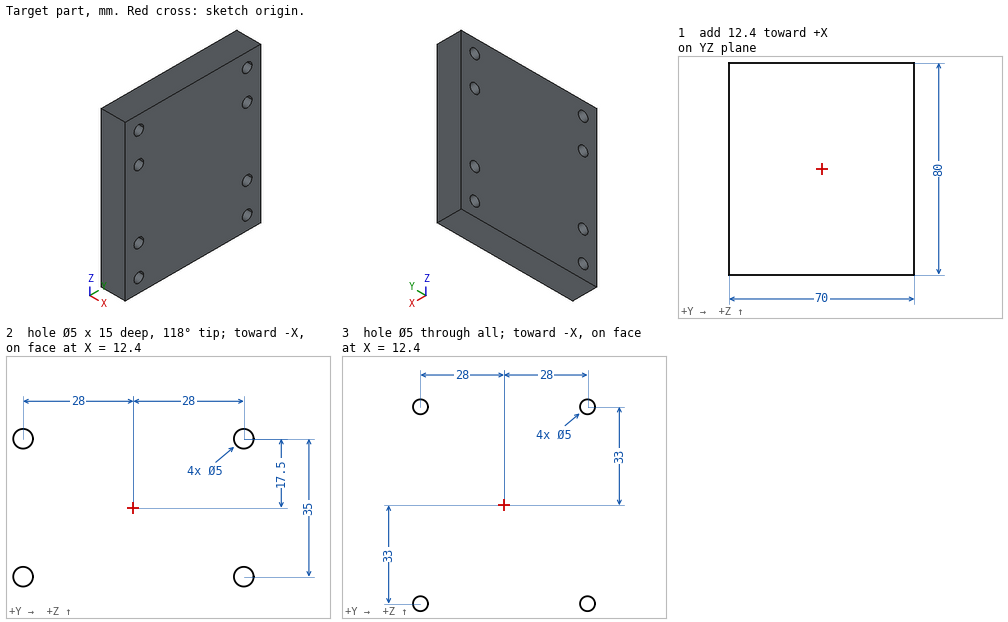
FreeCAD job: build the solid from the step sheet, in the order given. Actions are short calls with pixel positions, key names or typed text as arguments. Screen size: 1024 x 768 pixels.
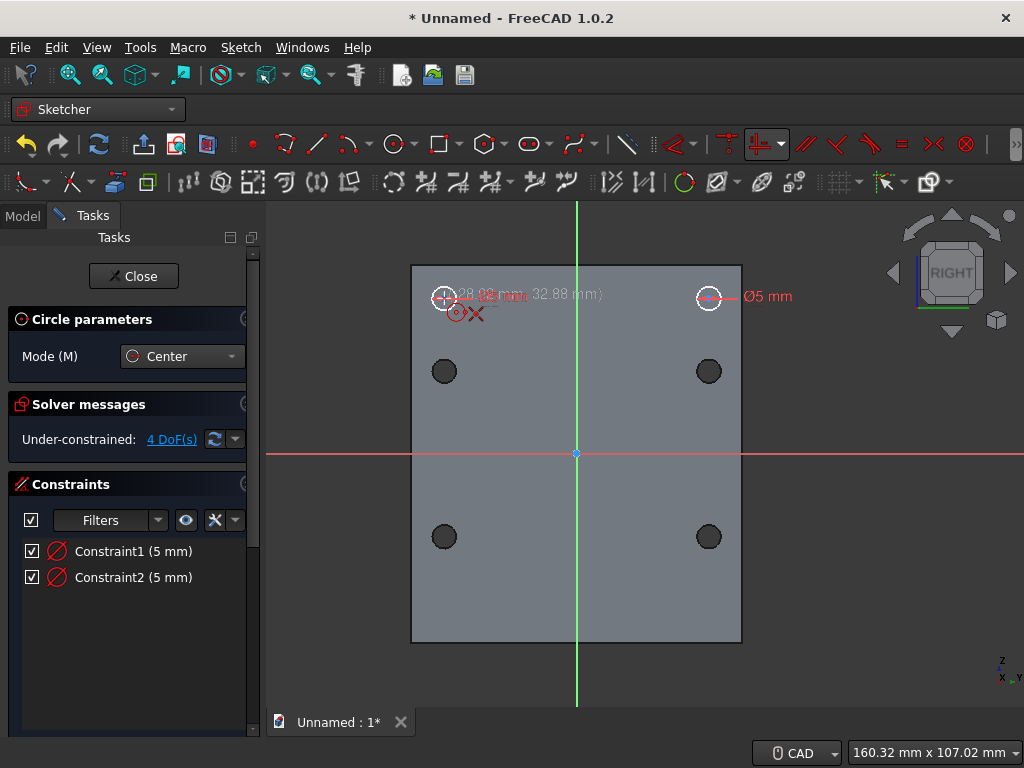
scroll(444, 610, up, 4)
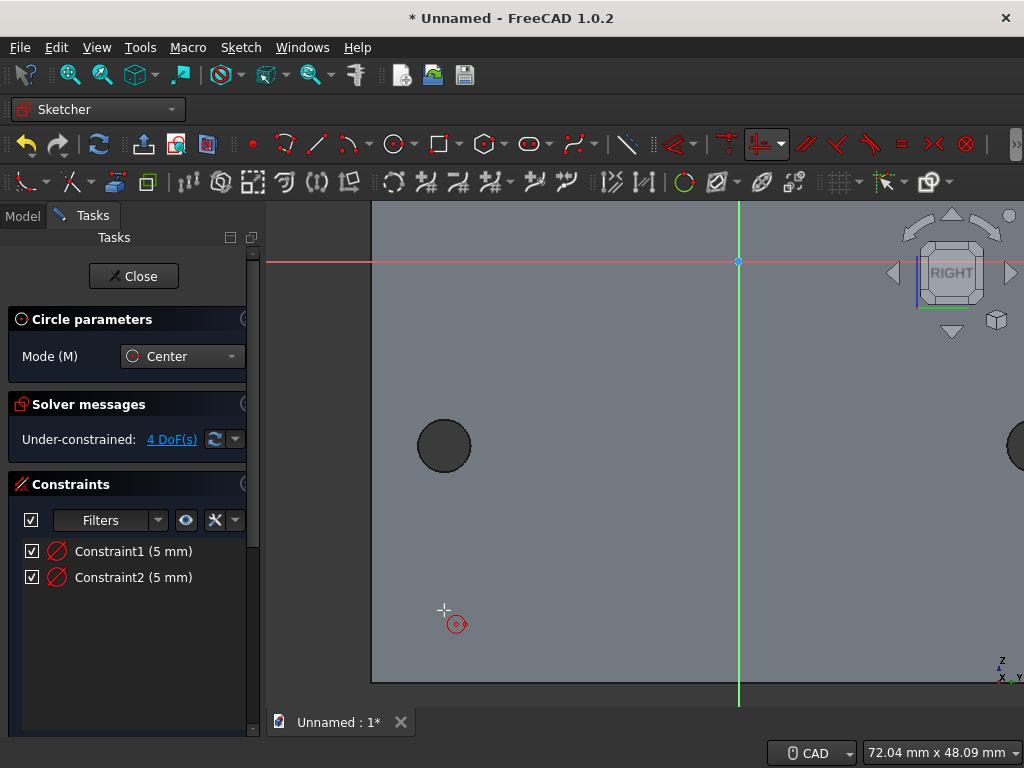
click(444, 609)
move(463, 590)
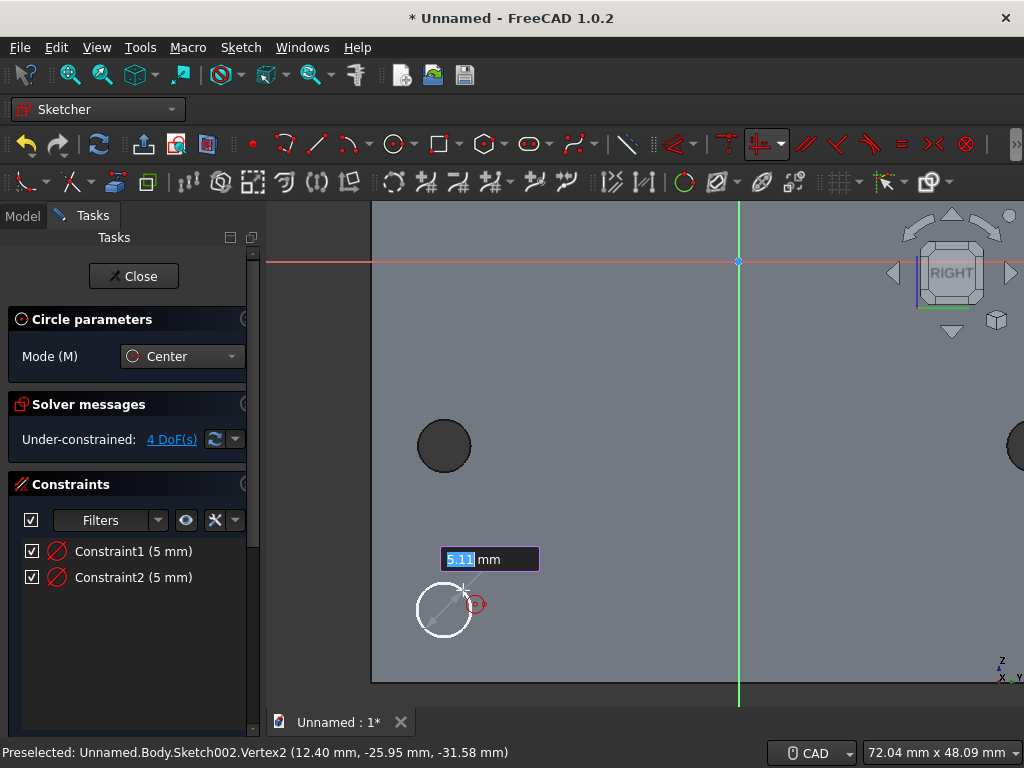
text(5)
key(Return)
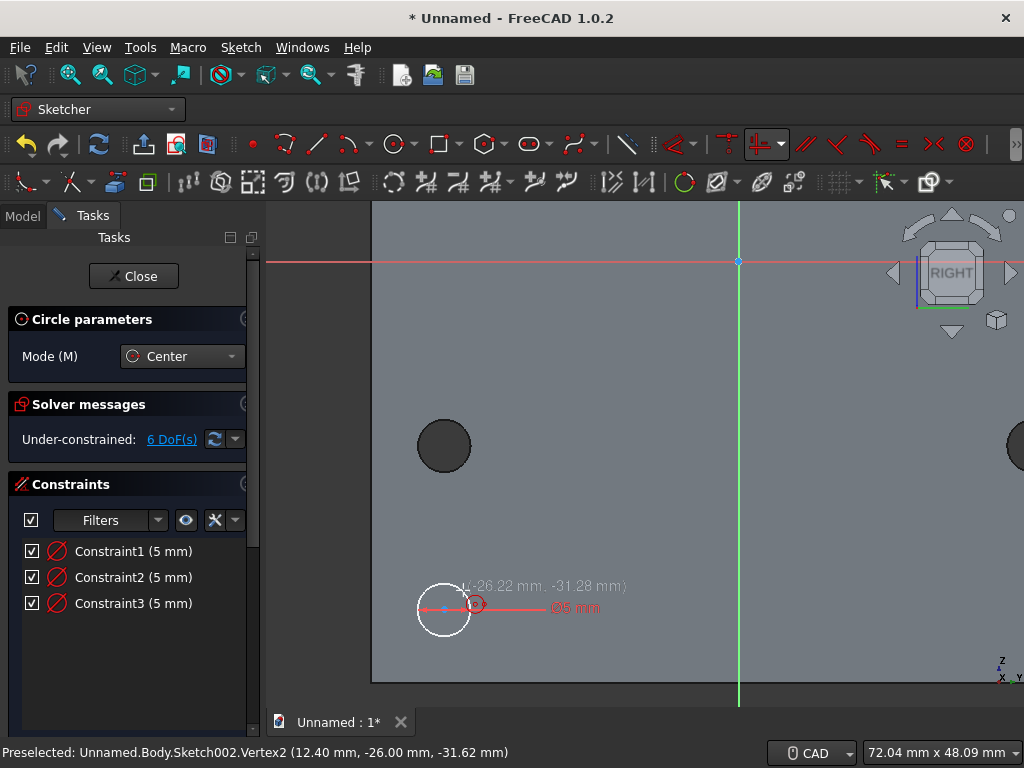
scroll(444, 611, down, 4)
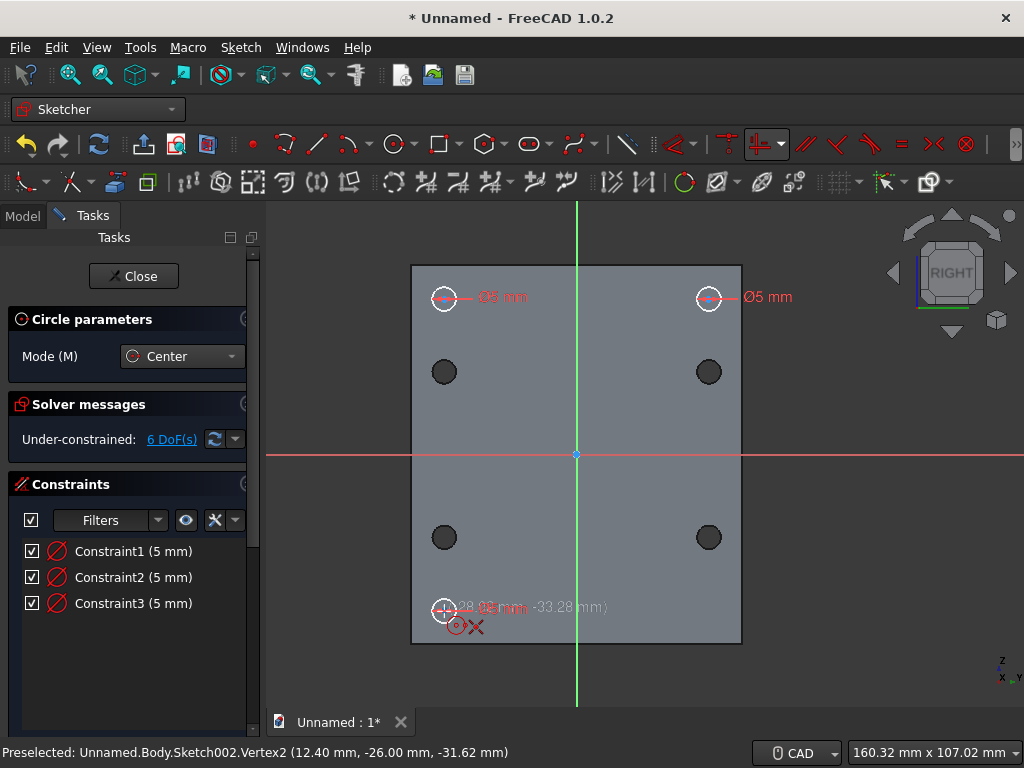
scroll(709, 611, up, 4)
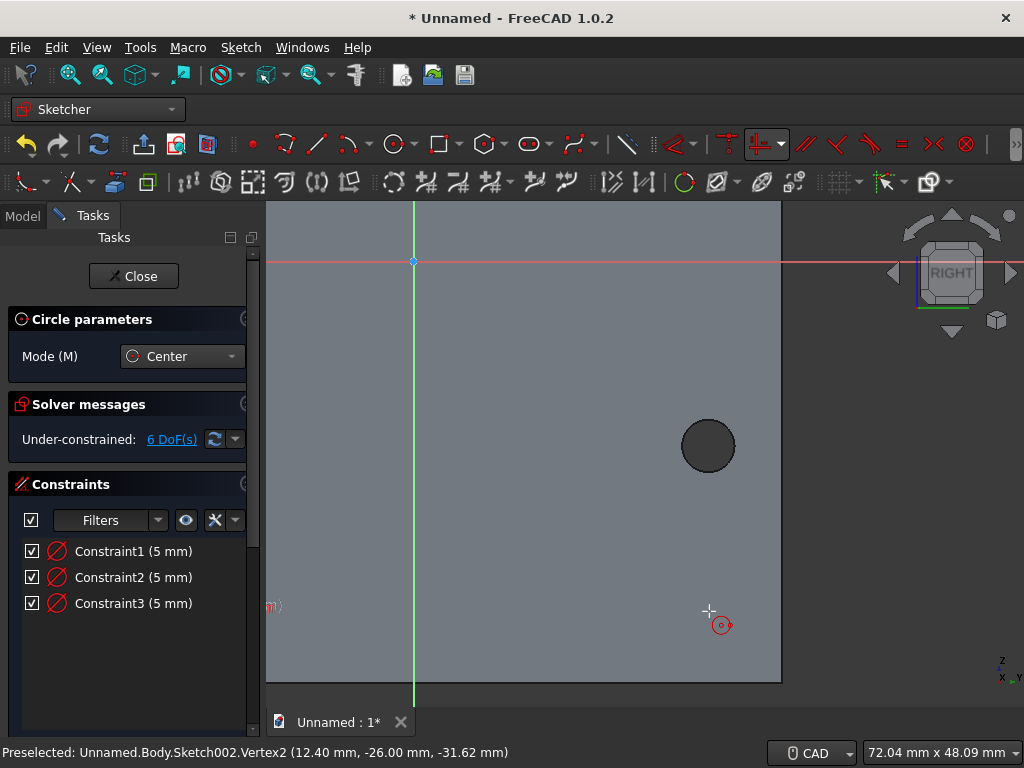
click(708, 609)
move(727, 590)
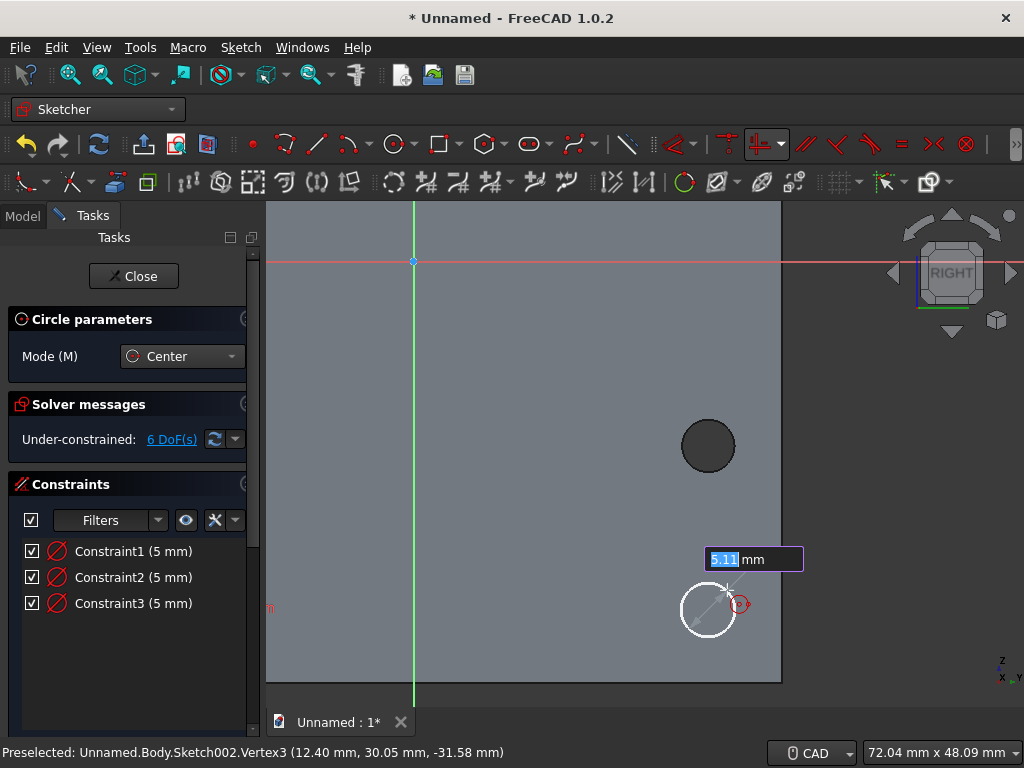
text(5)
key(Return)
key(Escape)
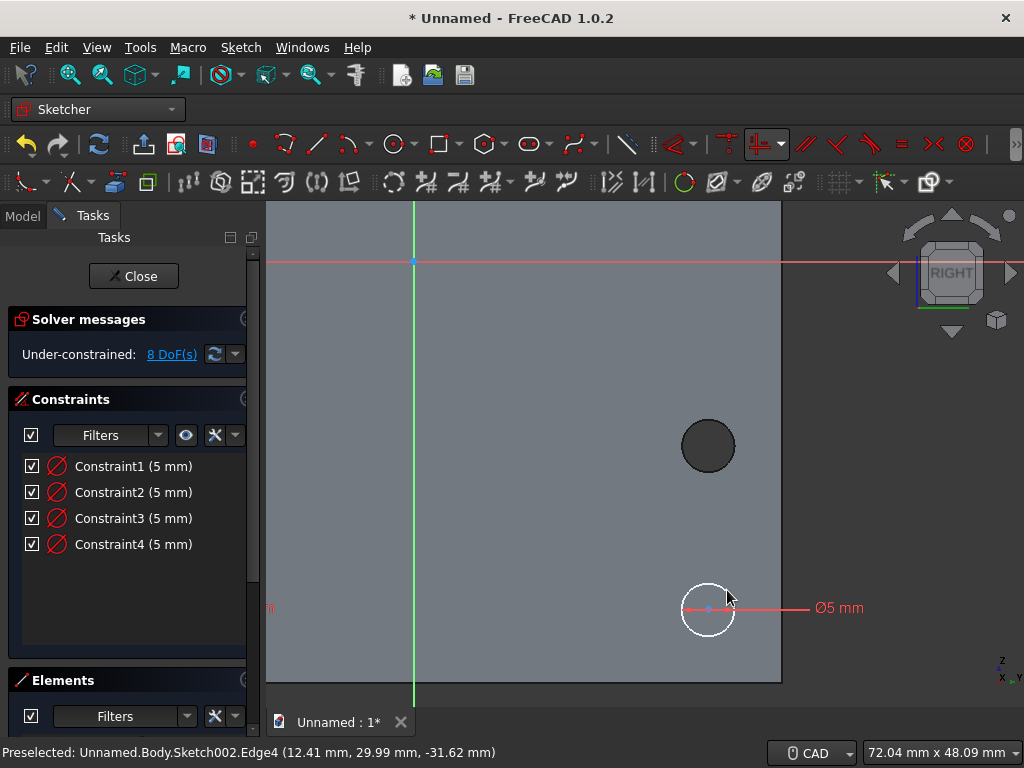
scroll(709, 611, down, 4)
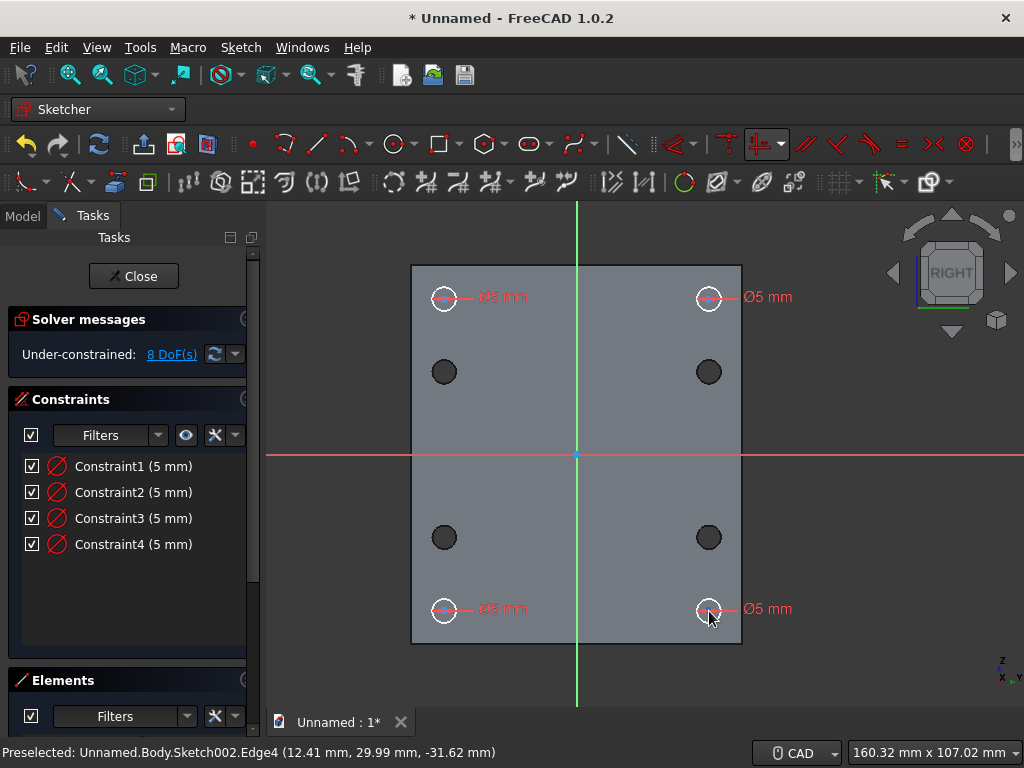
click(709, 299)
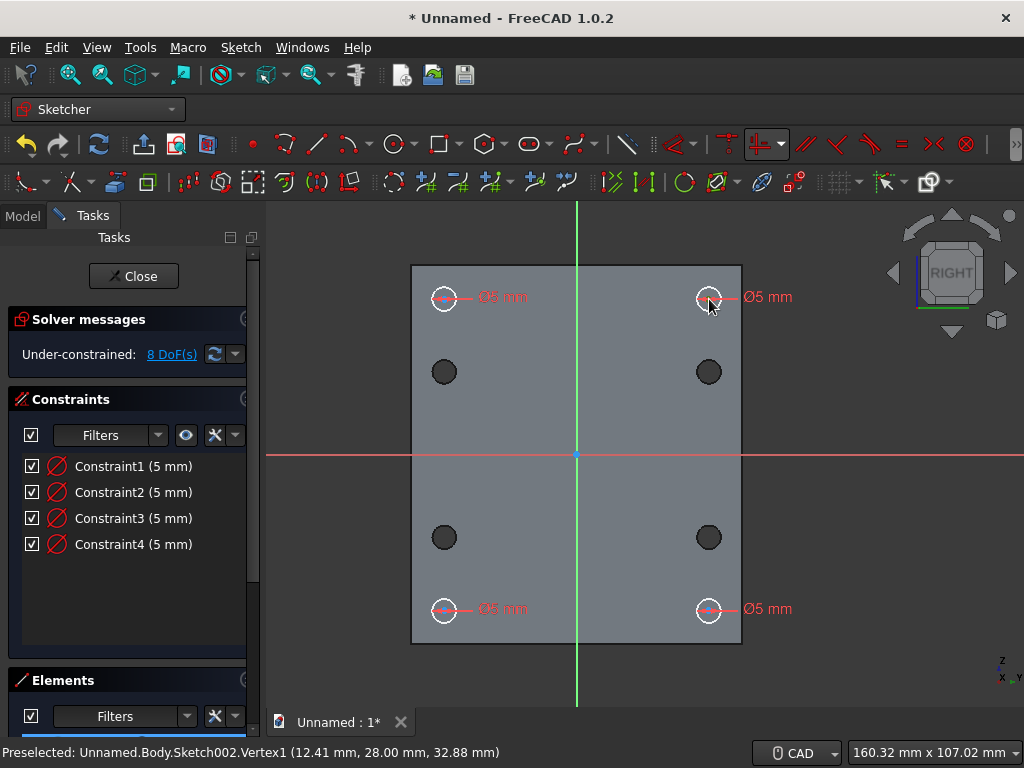
click(444, 299)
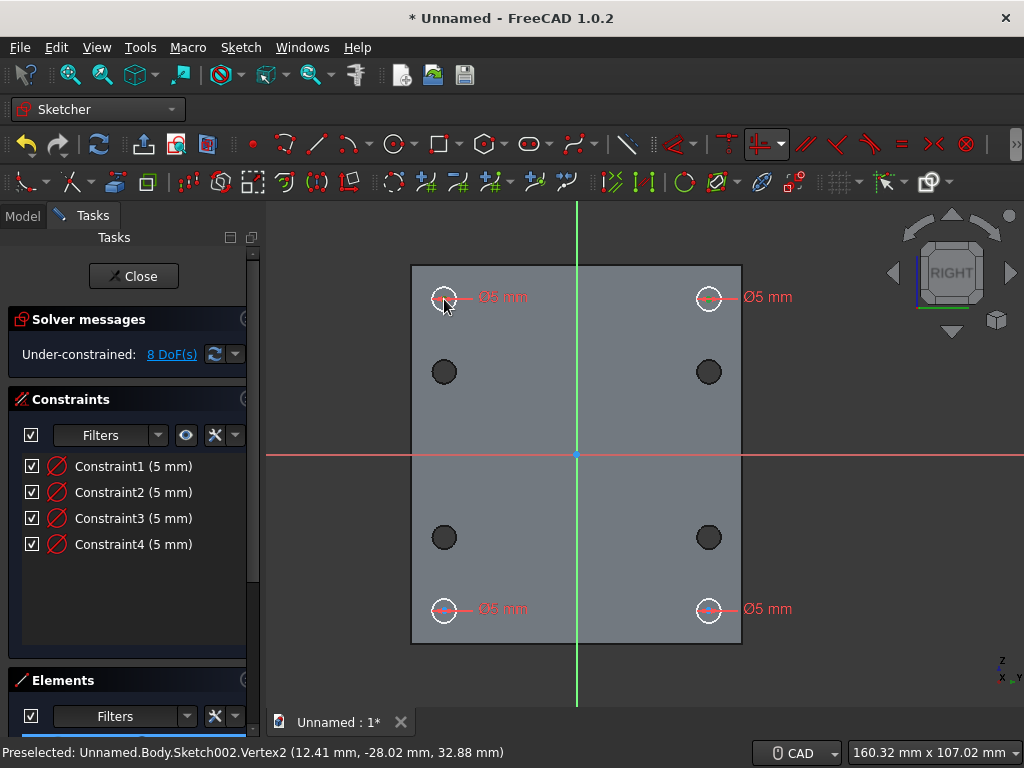
click(784, 144)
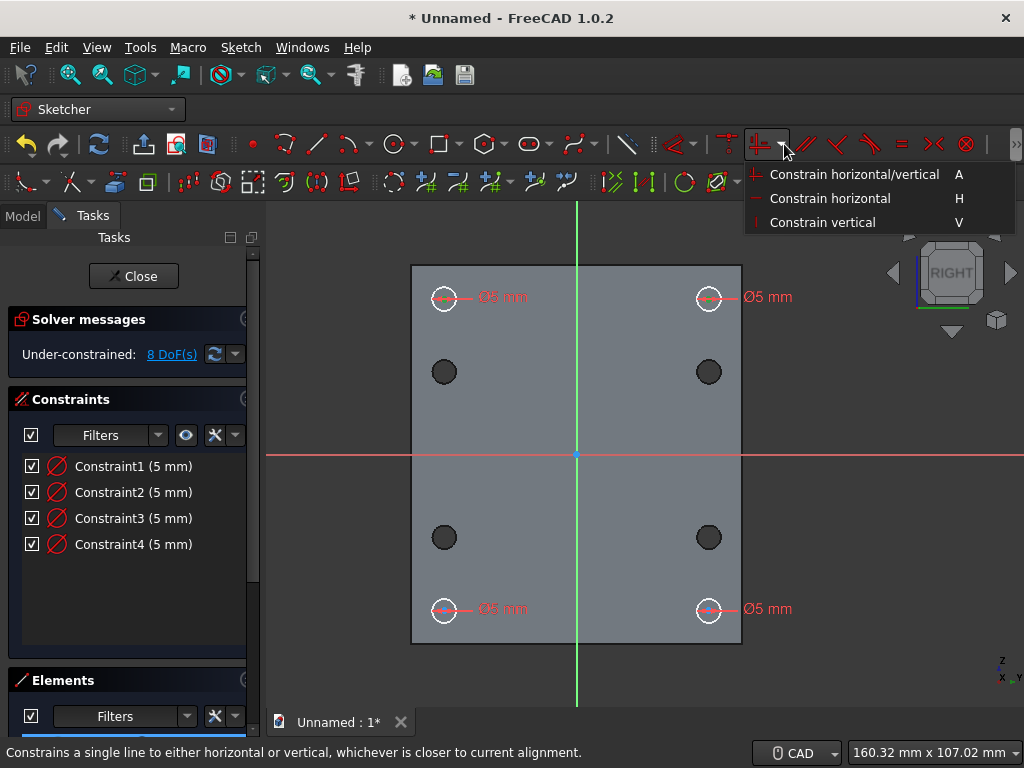
click(880, 198)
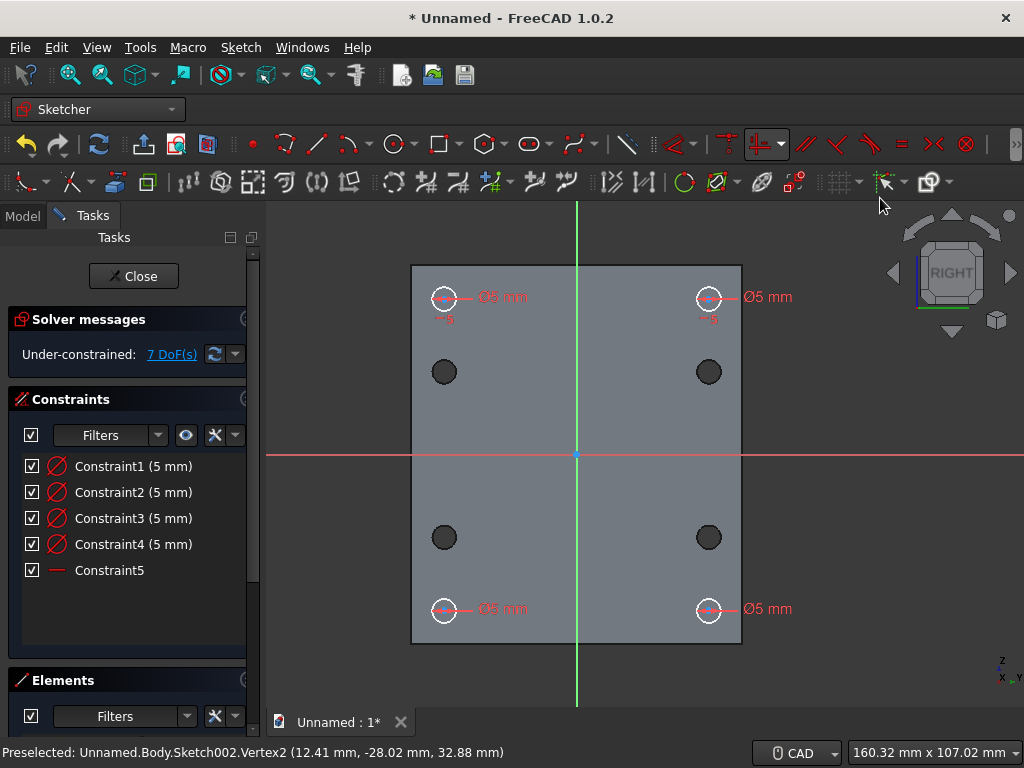
click(444, 299)